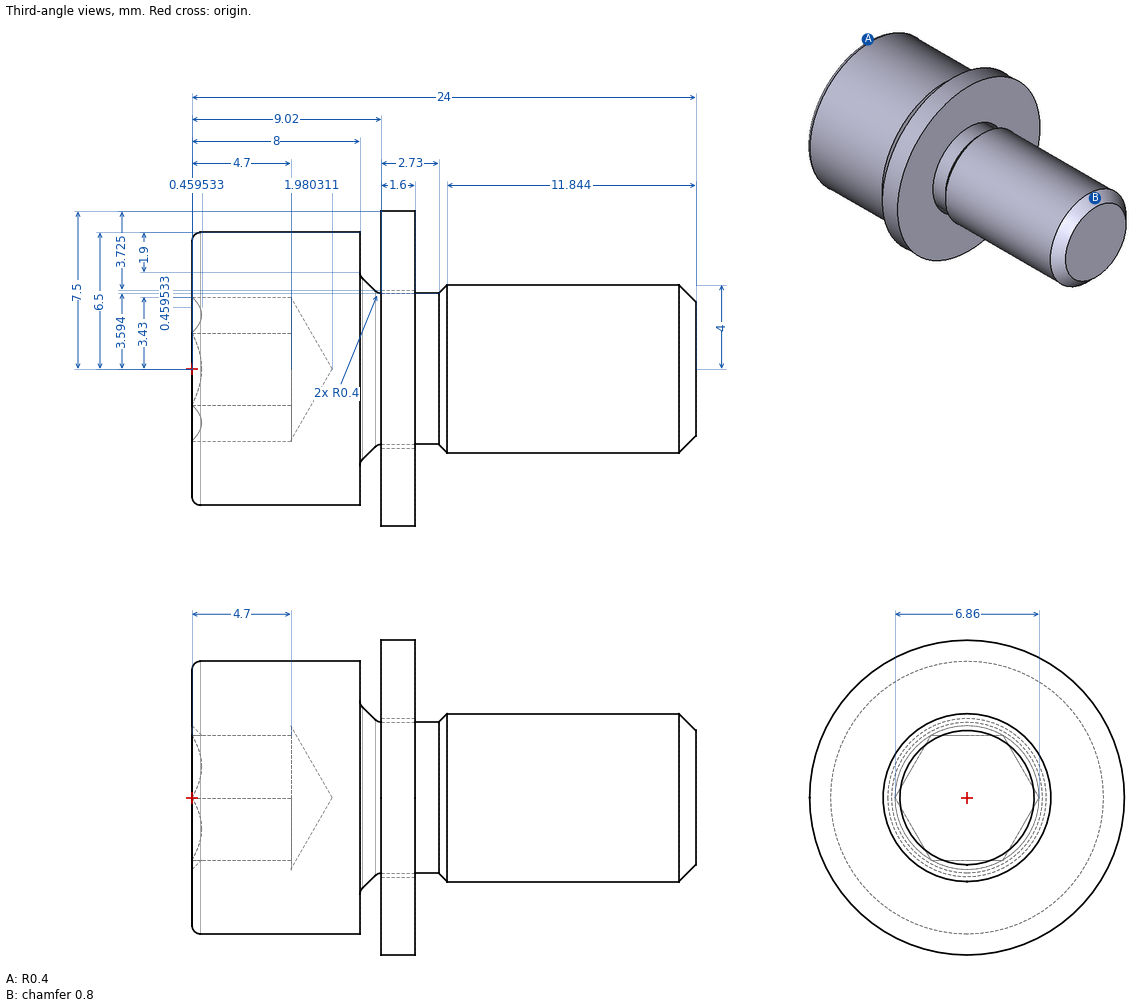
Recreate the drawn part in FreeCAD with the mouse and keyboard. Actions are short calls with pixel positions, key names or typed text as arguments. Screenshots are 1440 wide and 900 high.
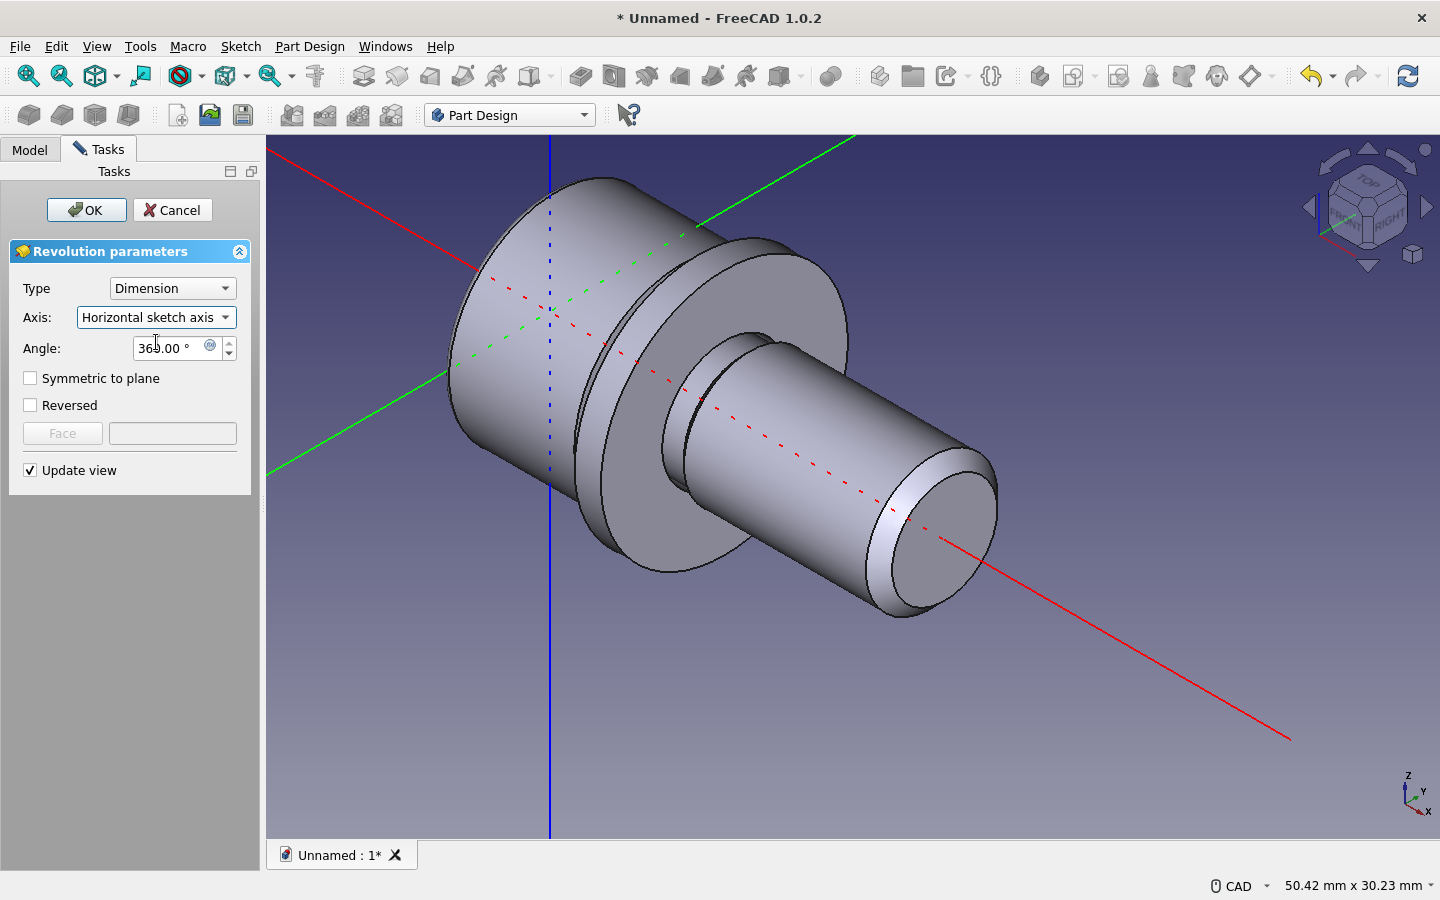
click(87, 210)